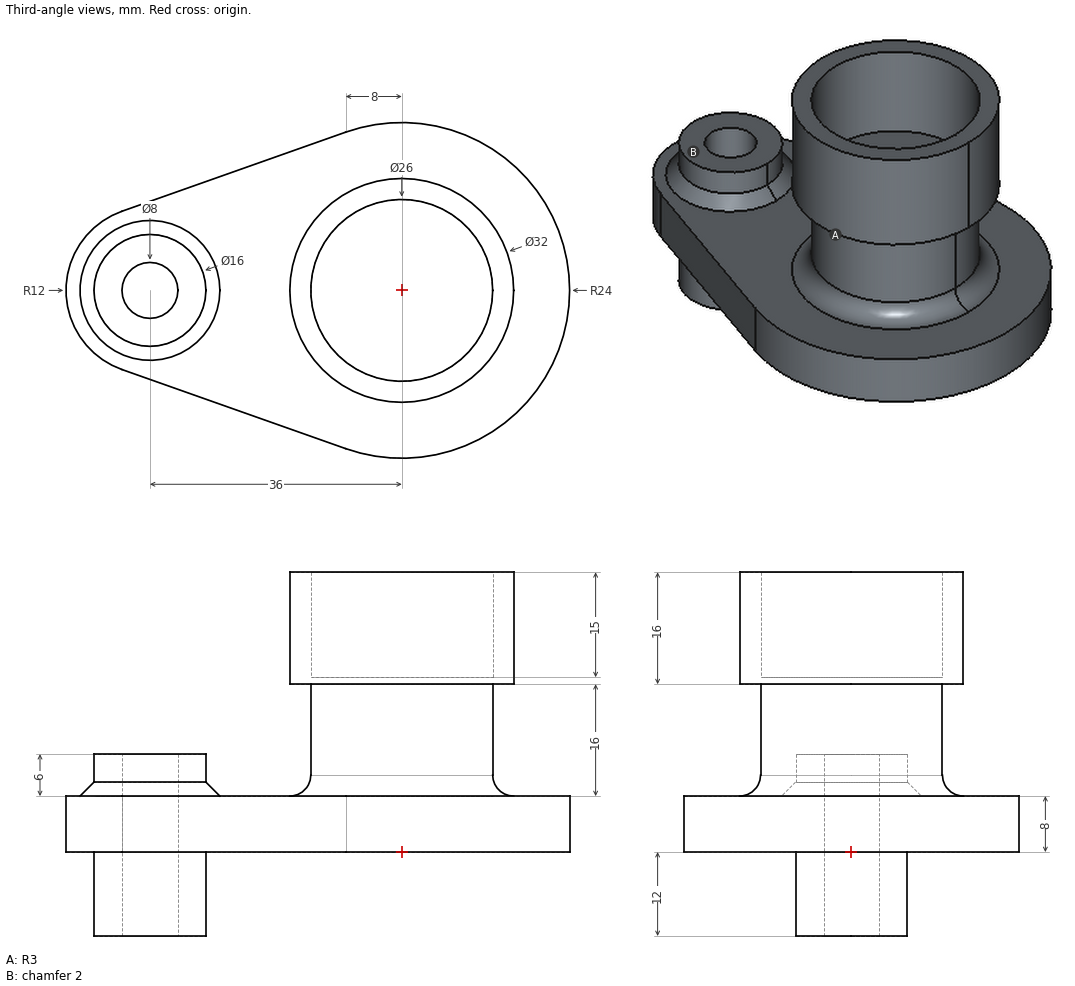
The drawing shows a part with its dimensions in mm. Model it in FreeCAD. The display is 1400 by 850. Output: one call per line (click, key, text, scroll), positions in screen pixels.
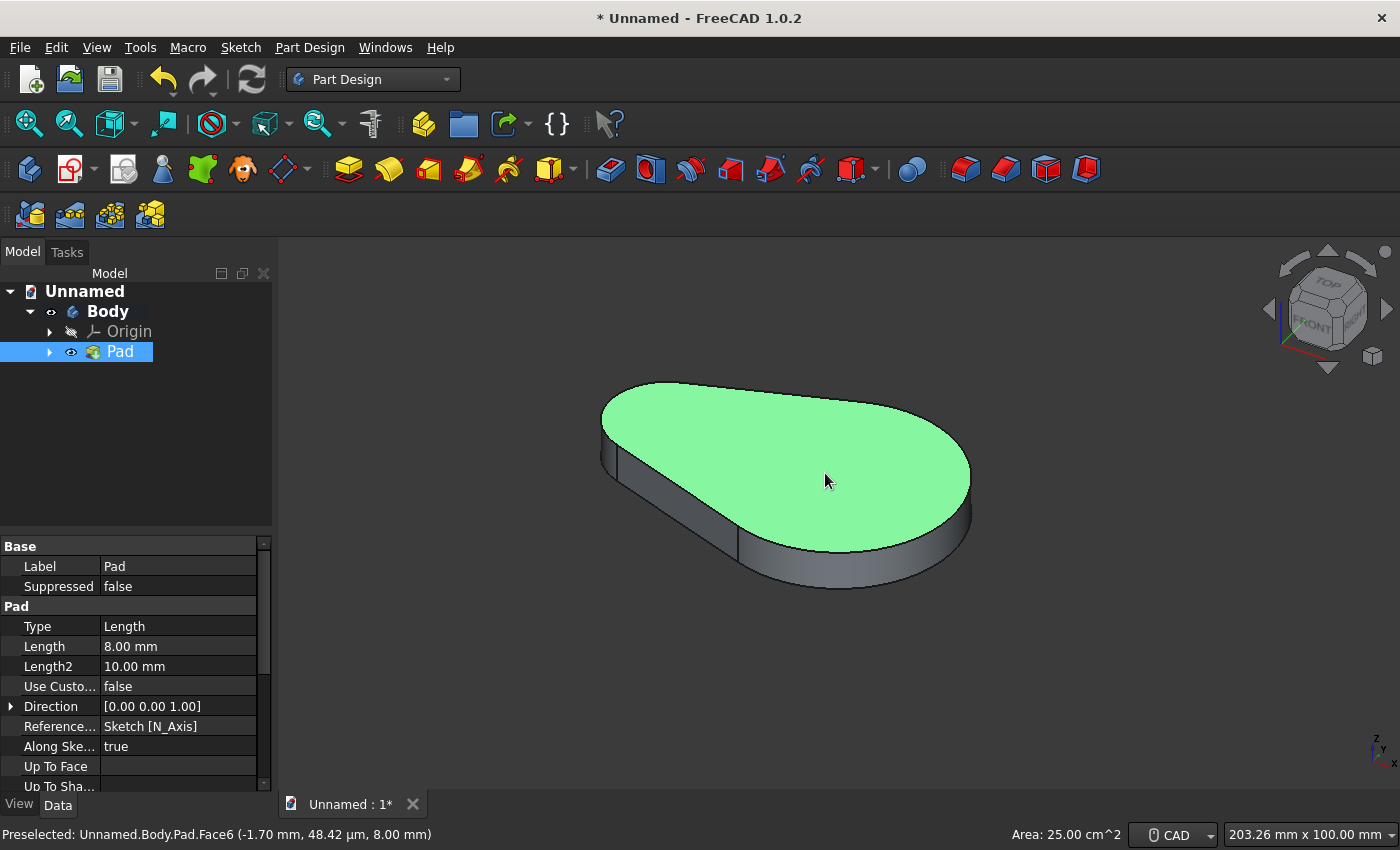
click(70, 170)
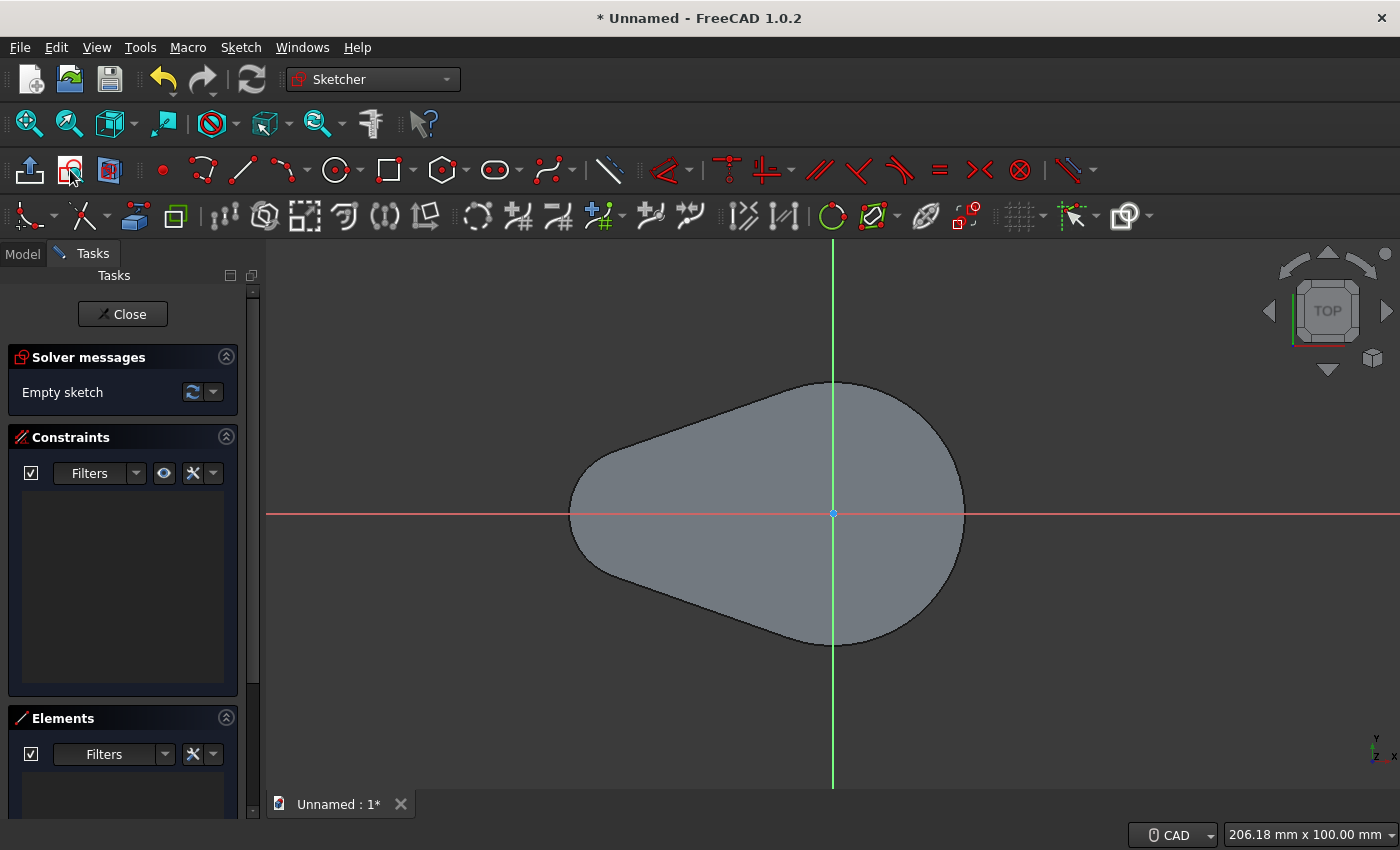
scroll(593, 514, up, 7)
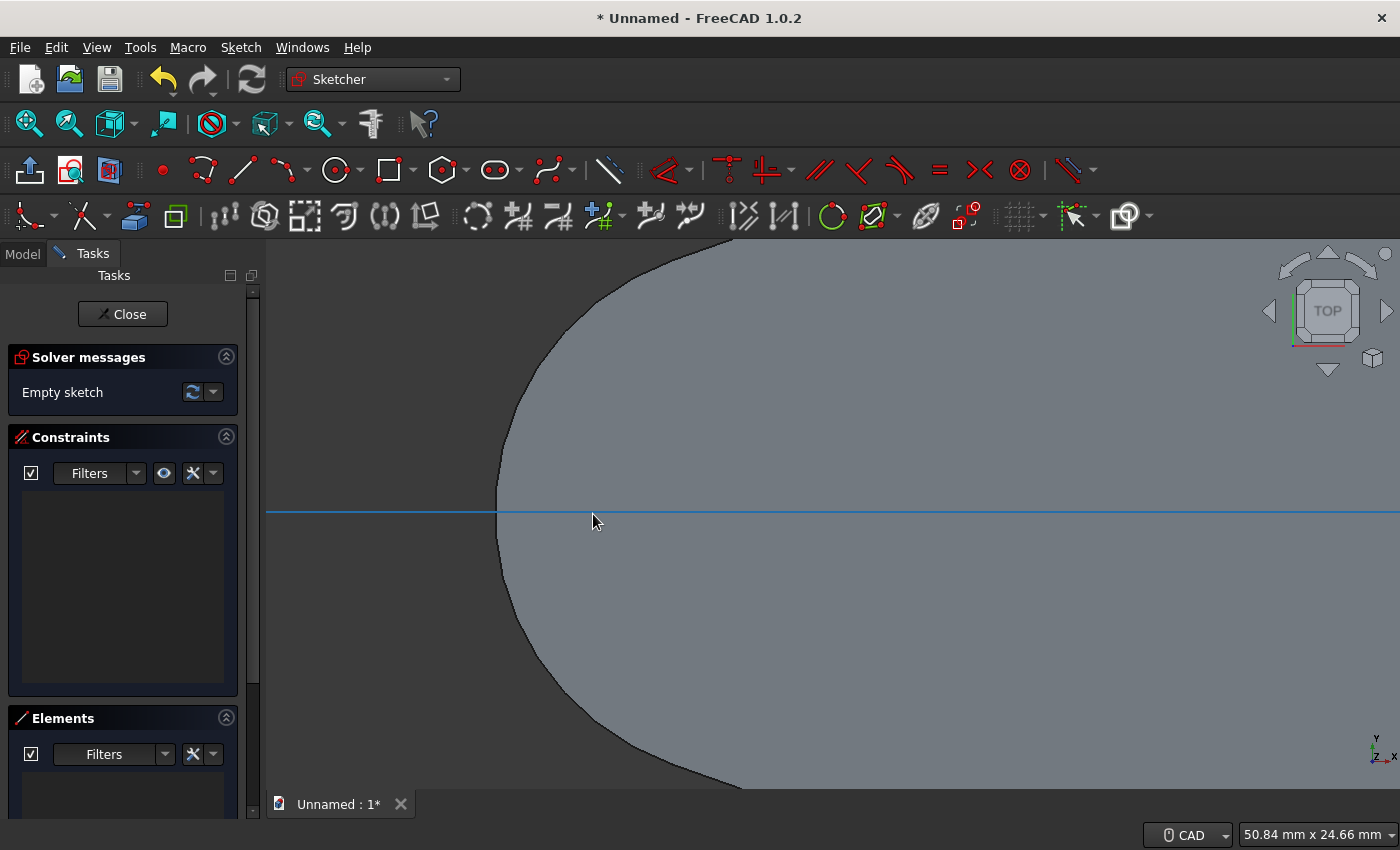
key(g)
key(c)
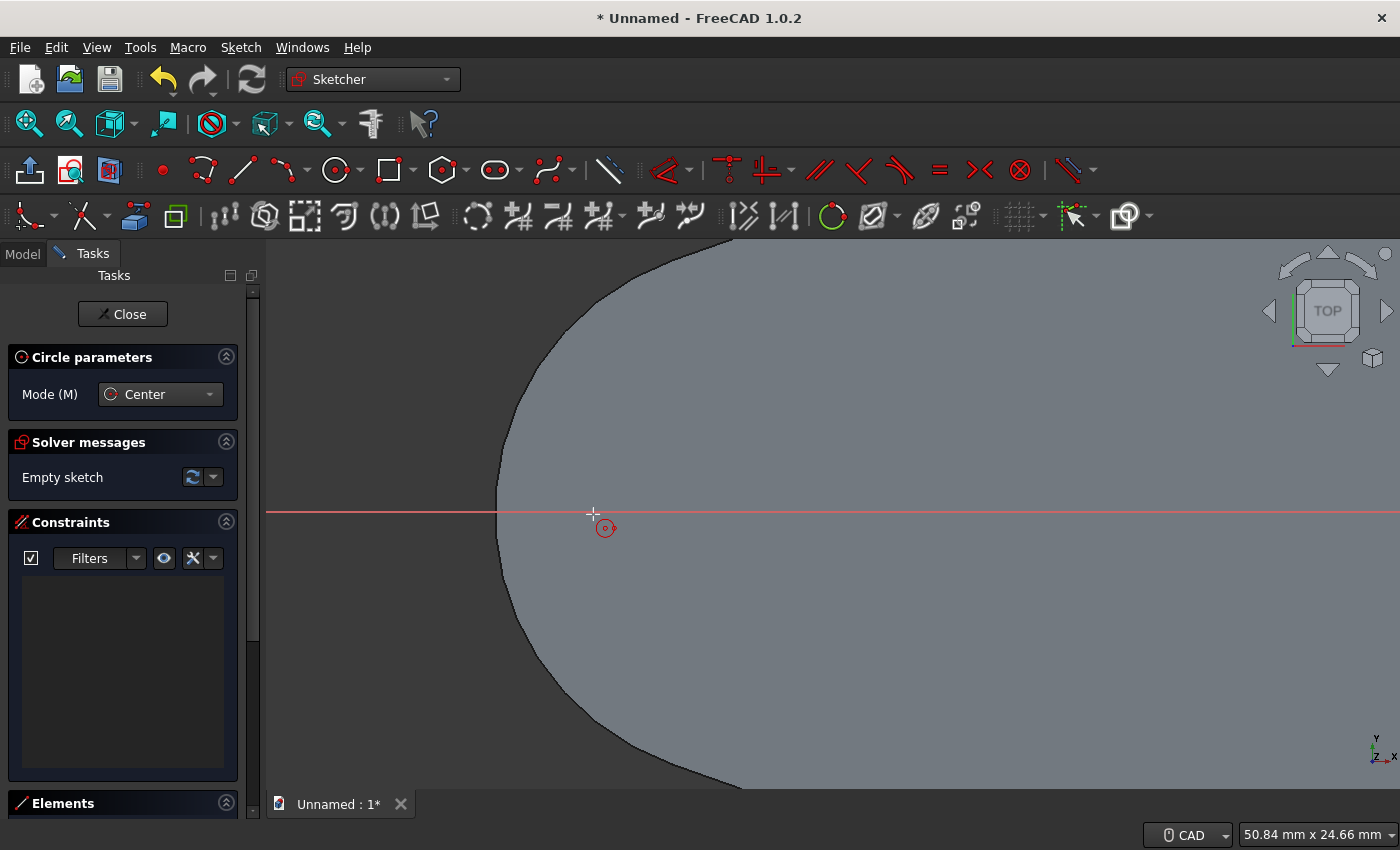
click(762, 512)
move(889, 386)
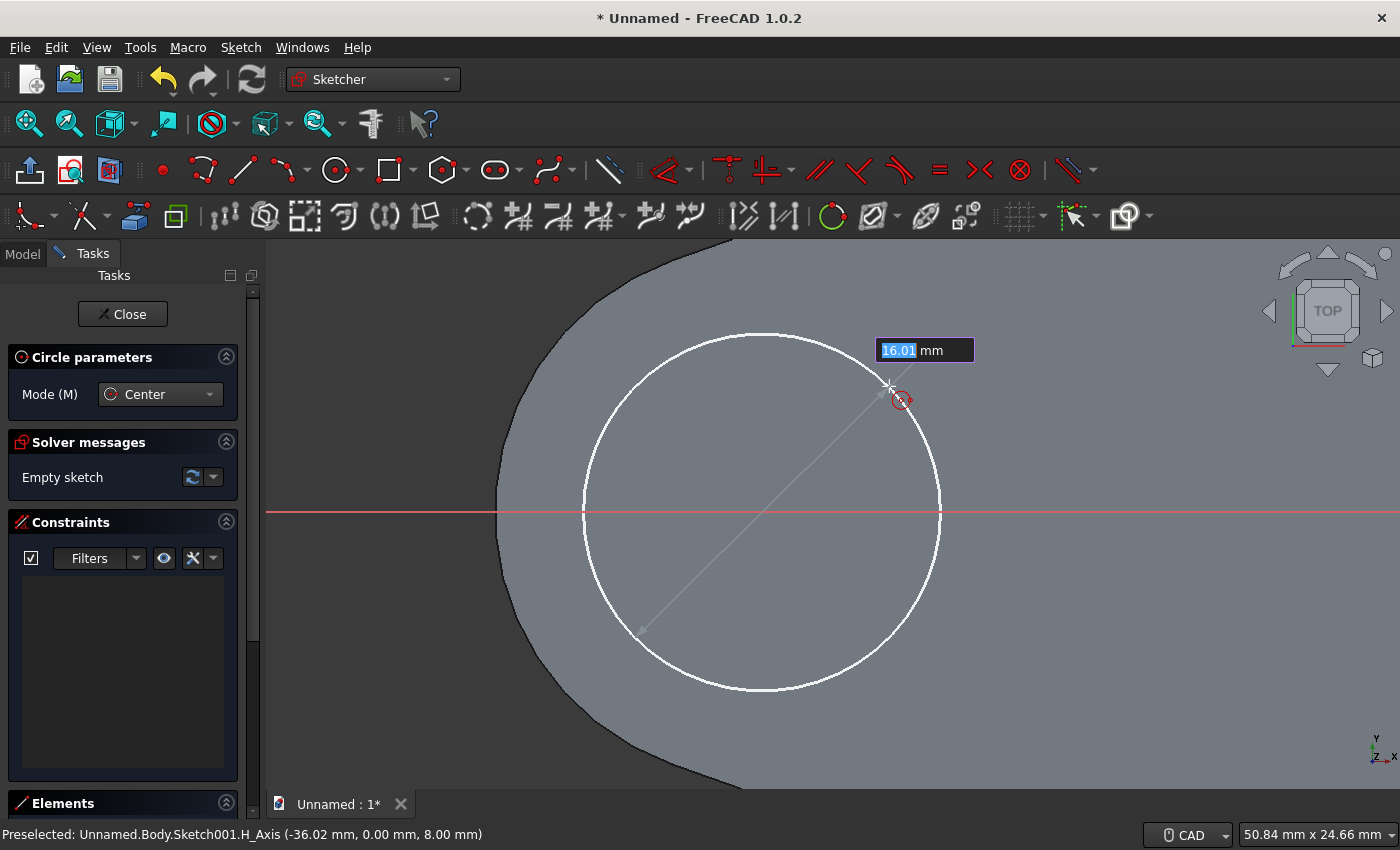
text(16)
key(Return)
key(Escape)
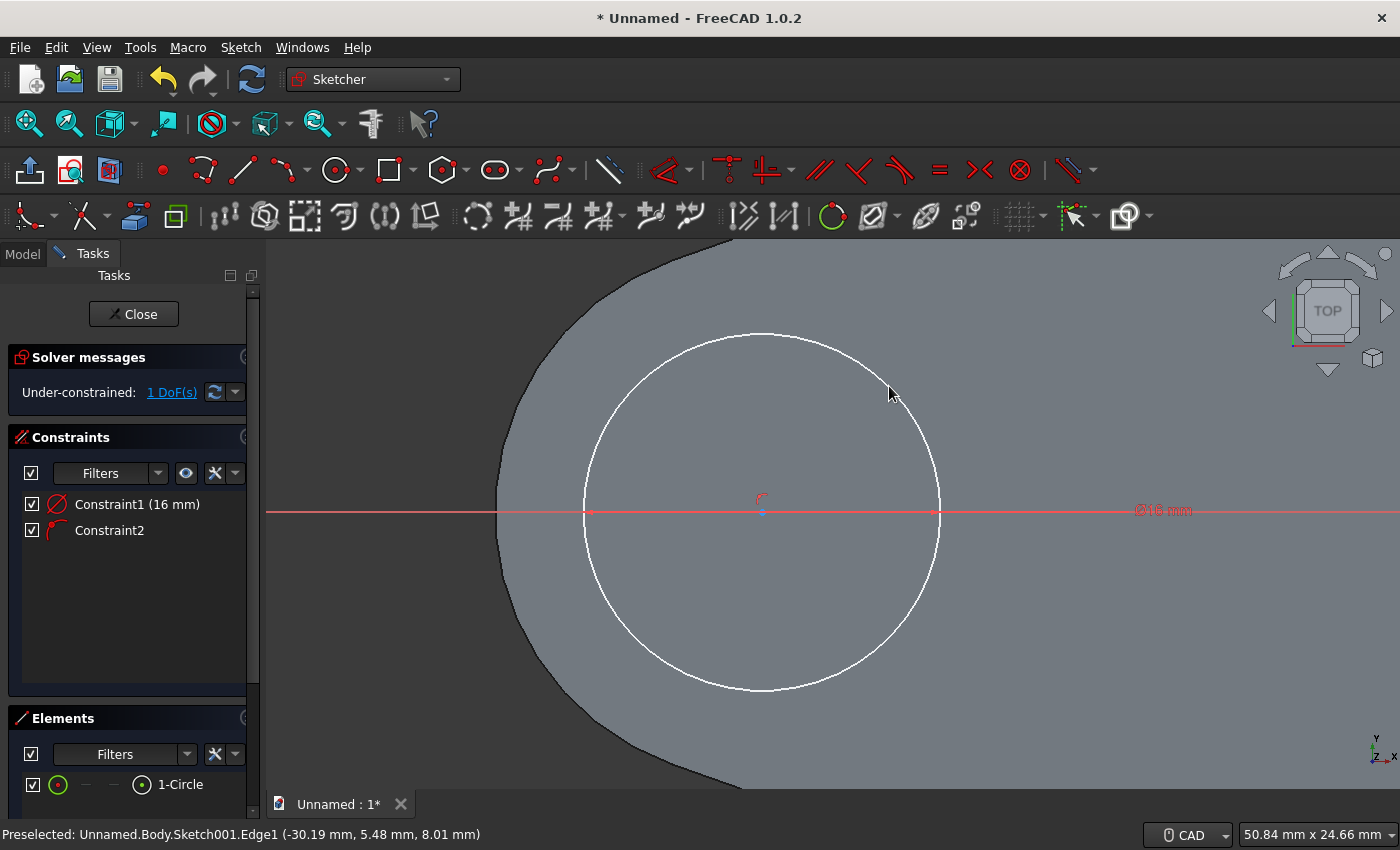
click(664, 170)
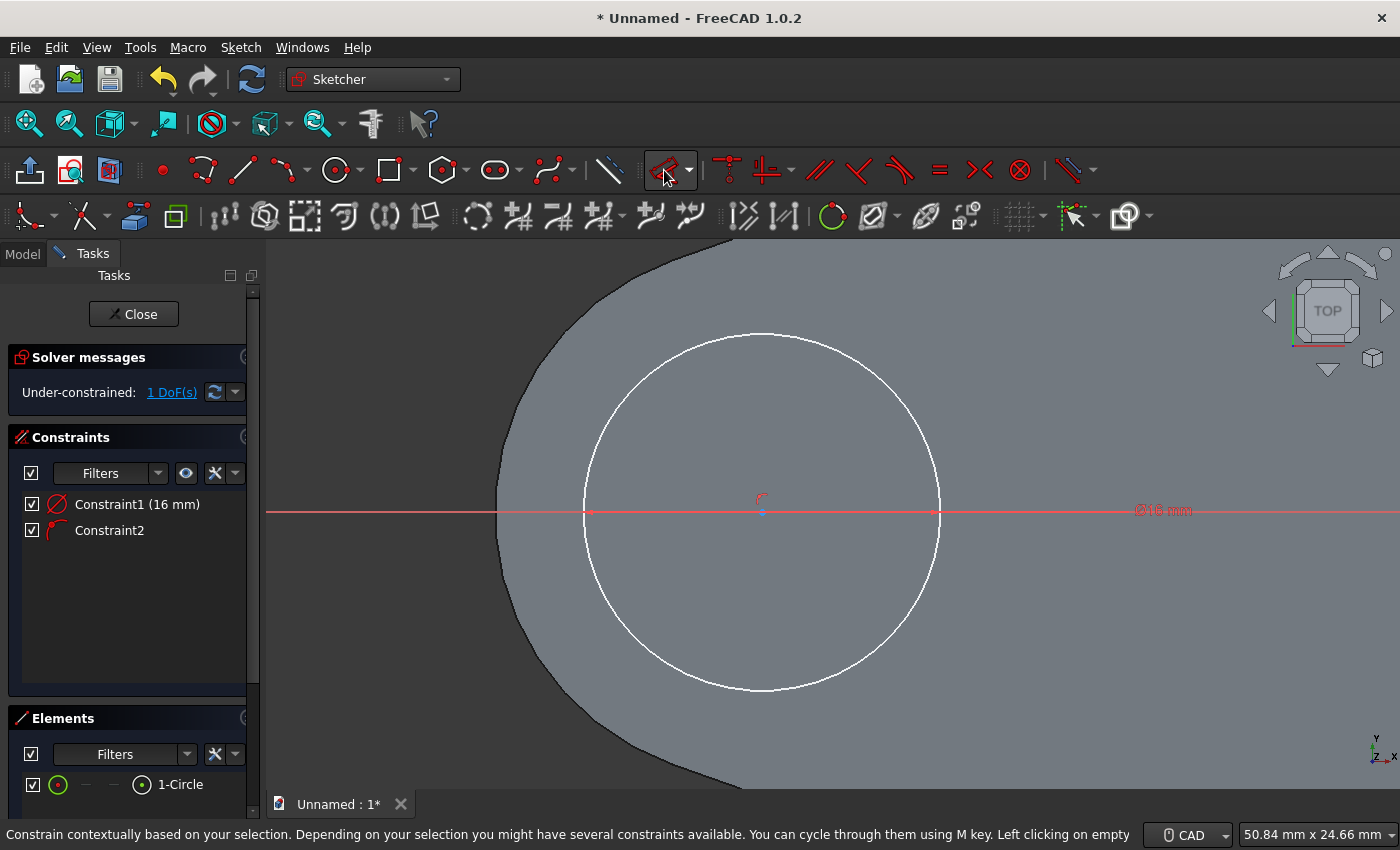
click(762, 512)
click(999, 546)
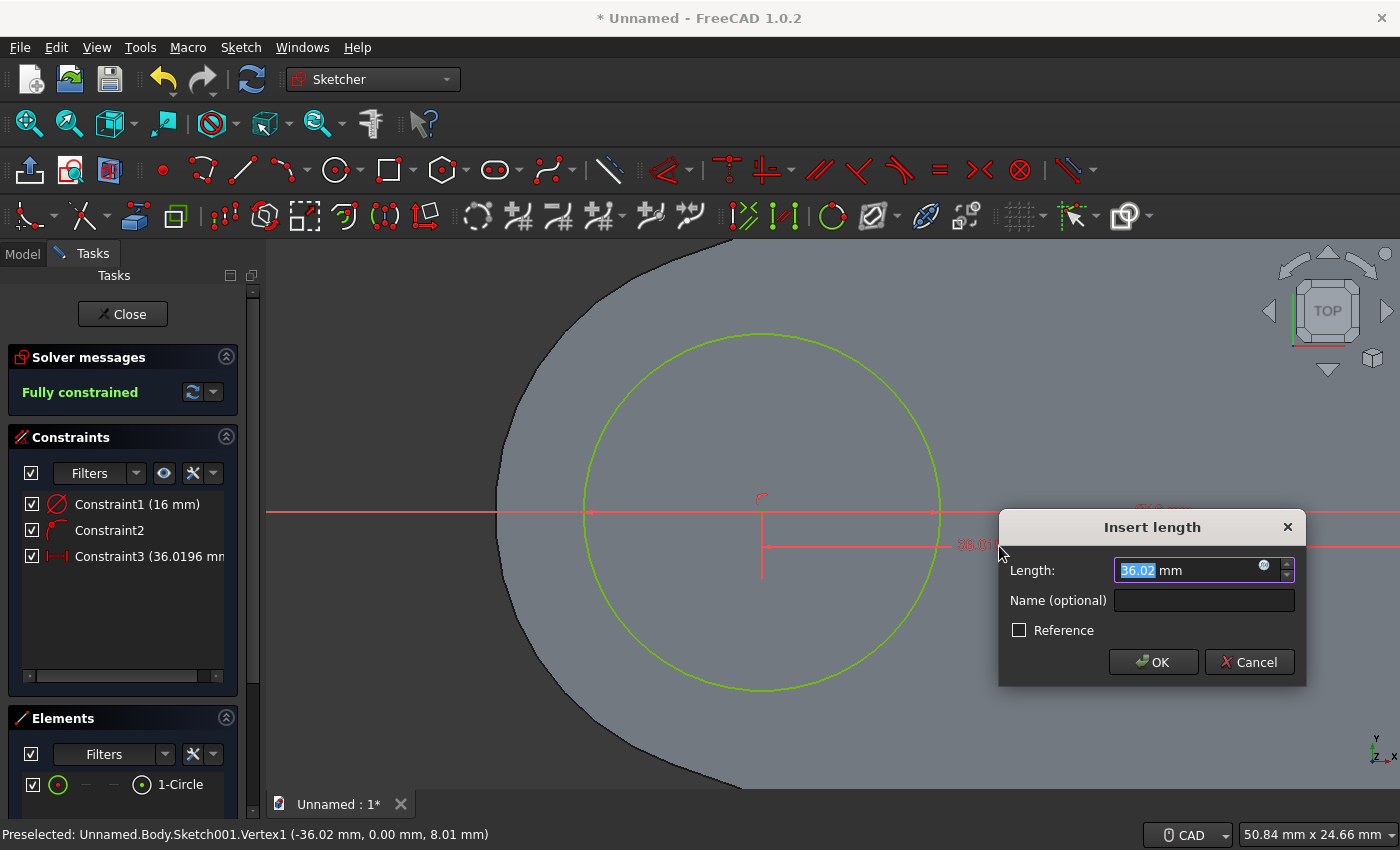
text(36)
key(Return)
key(Escape)